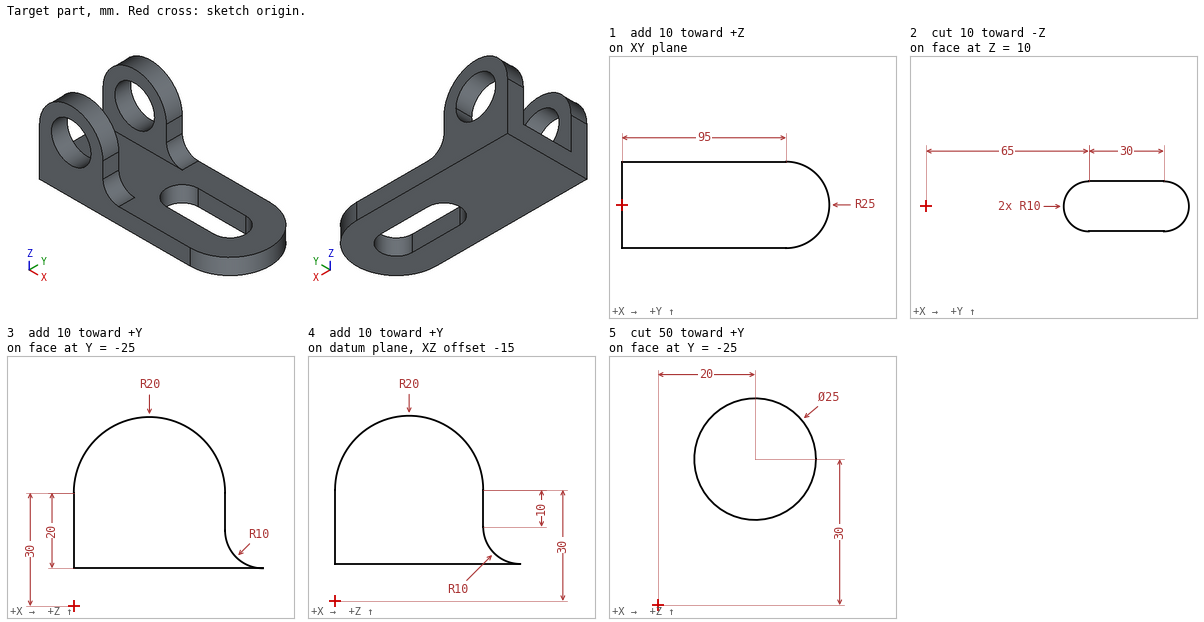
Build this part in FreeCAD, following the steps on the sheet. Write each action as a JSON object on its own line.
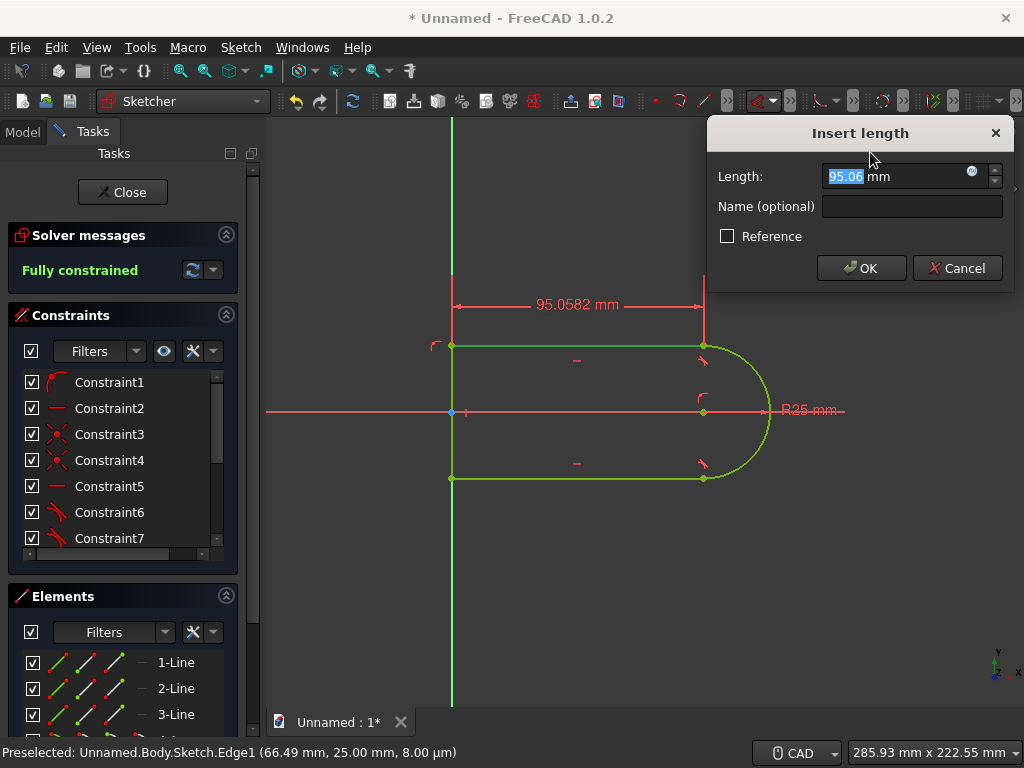
{"action": "type", "text": "95"}
{"action": "key", "text": "Return"}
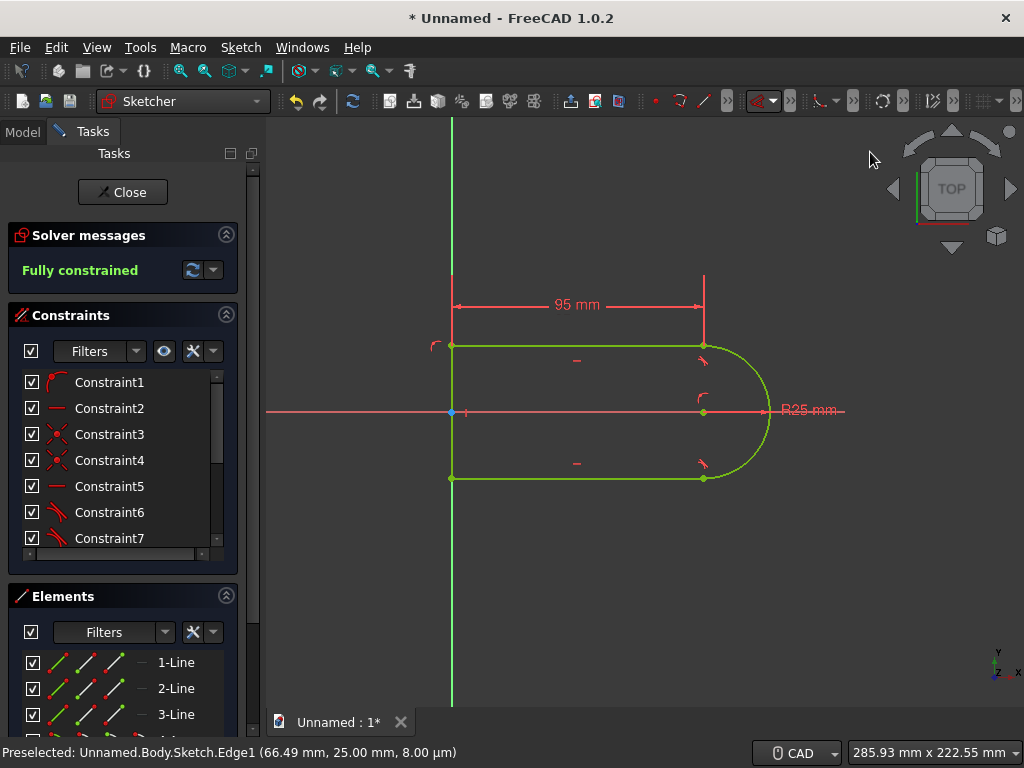
{"action": "left_click", "coordinate": [123, 192]}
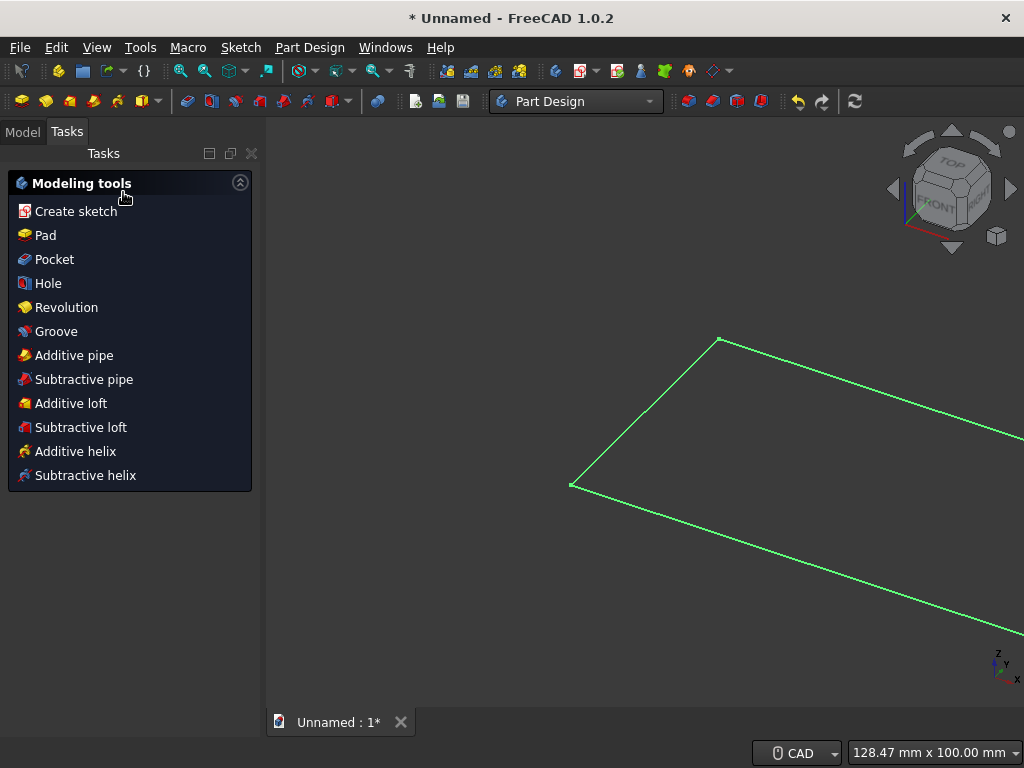
{"action": "left_click", "coordinate": [22, 102]}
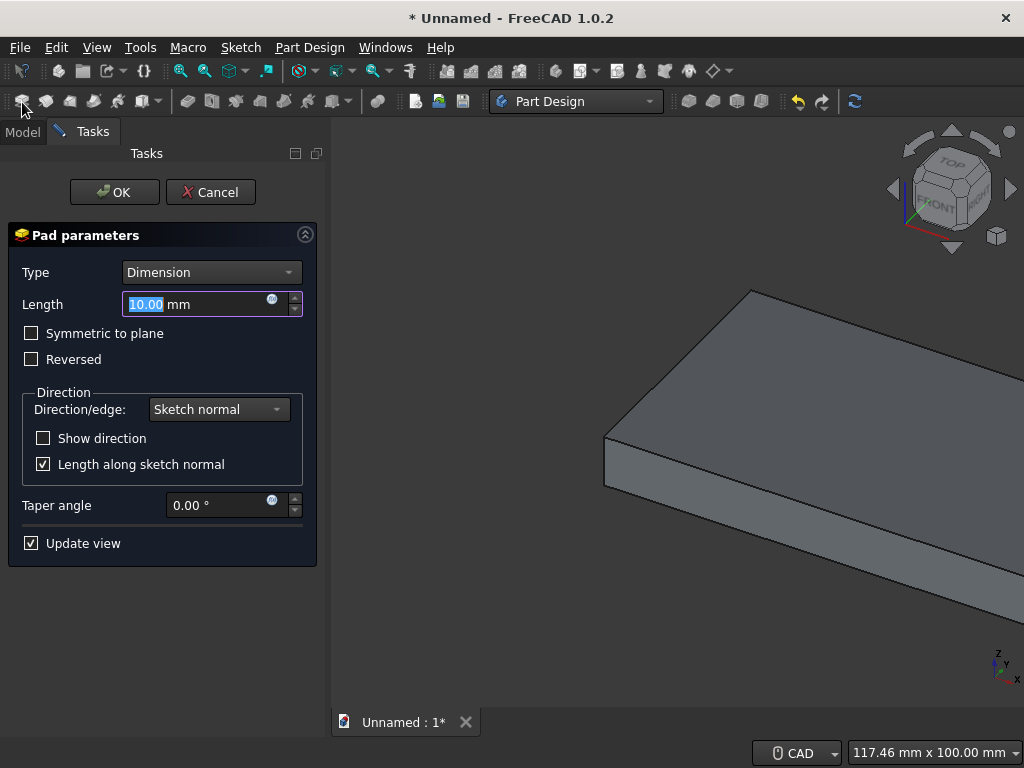
{"action": "type", "text": "10"}
{"action": "key", "text": "Tab"}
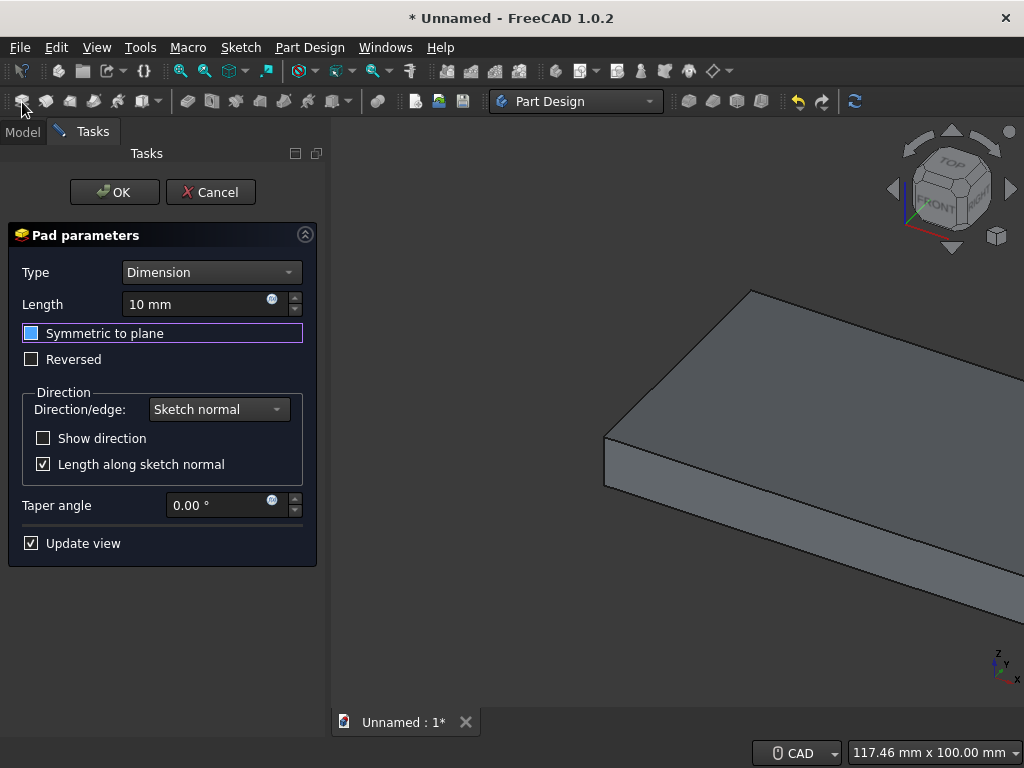
{"action": "left_click", "coordinate": [115, 192]}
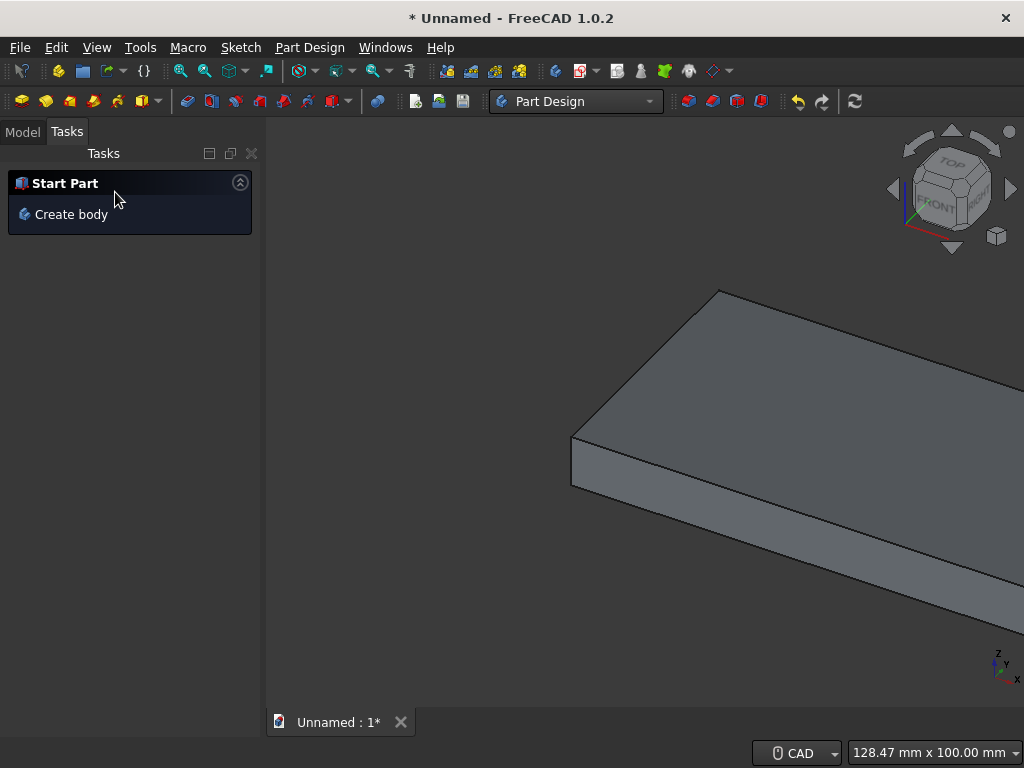
{"action": "left_click", "coordinate": [182, 72]}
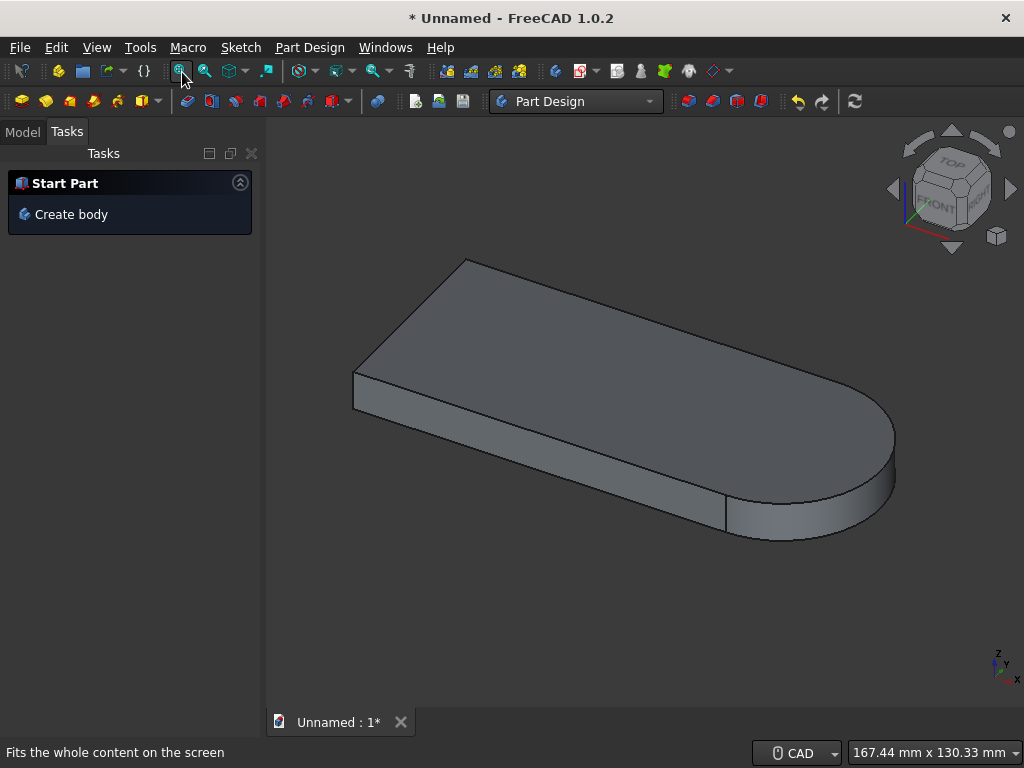
{"action": "left_click", "coordinate": [780, 437]}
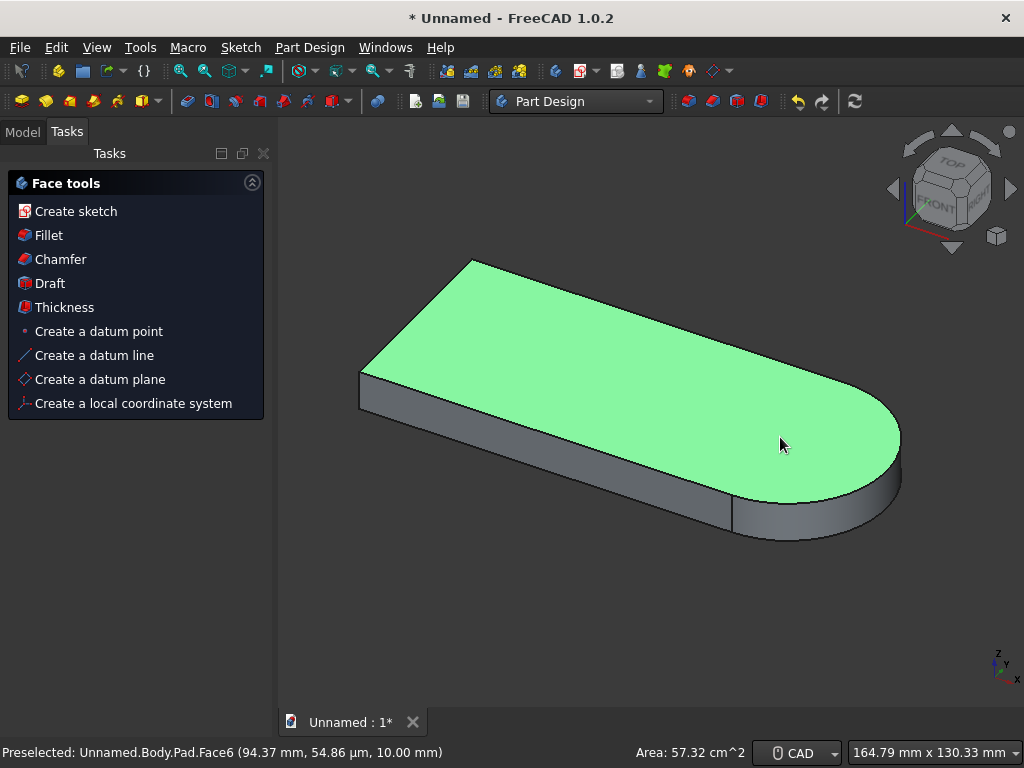
{"action": "left_click", "coordinate": [580, 72]}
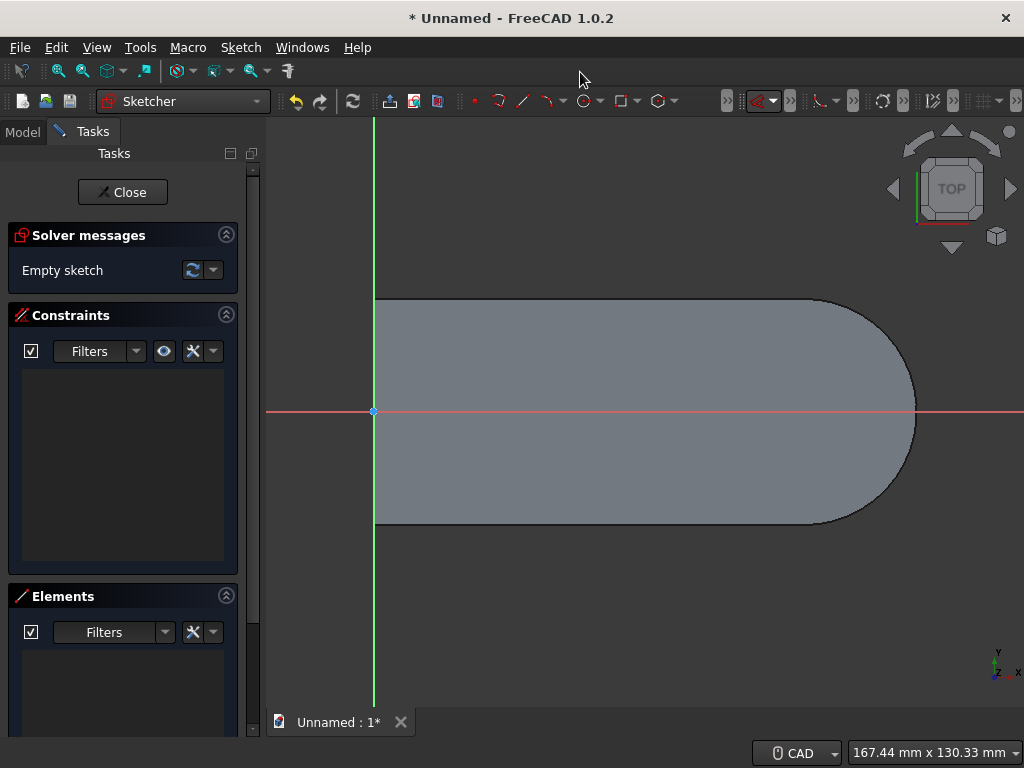
{"action": "scroll", "coordinate": [420, 412], "scroll_direction": "down", "scroll_amount": 1}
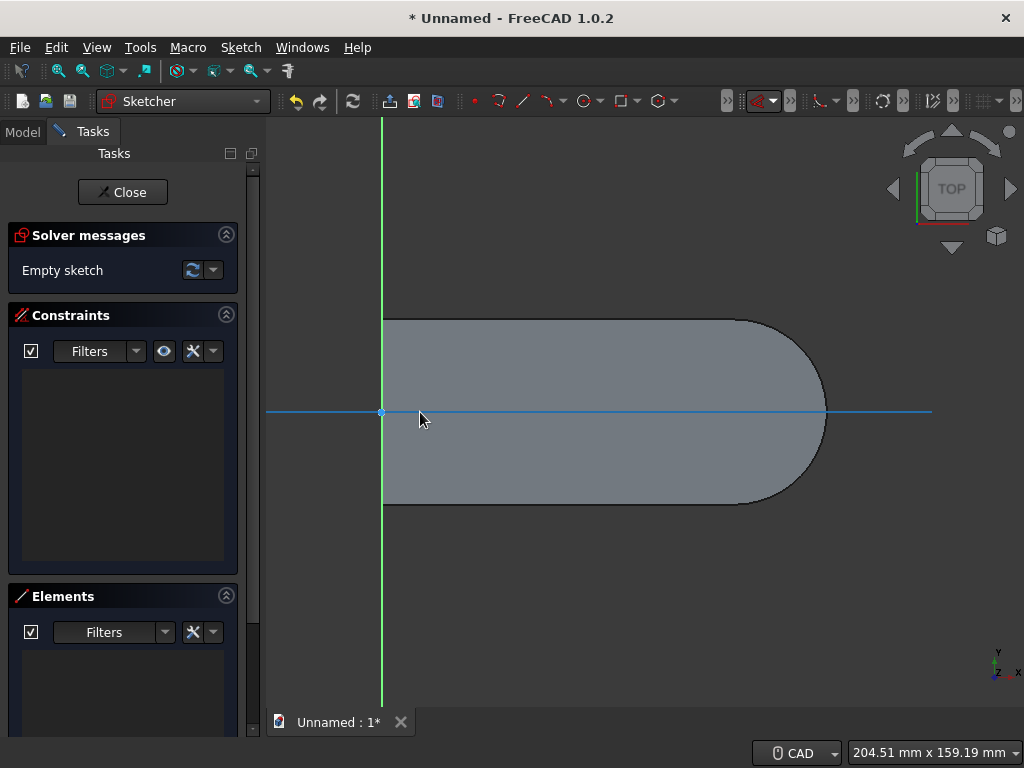
{"action": "key", "text": "g s"}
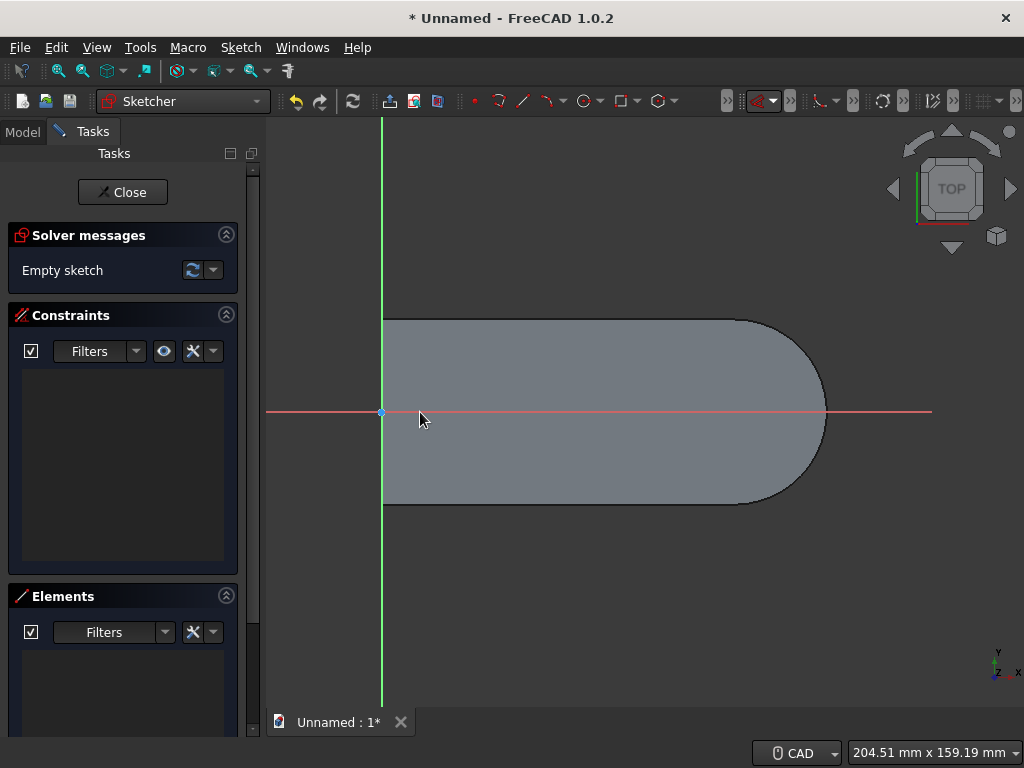
{"action": "left_click", "coordinate": [623, 412]}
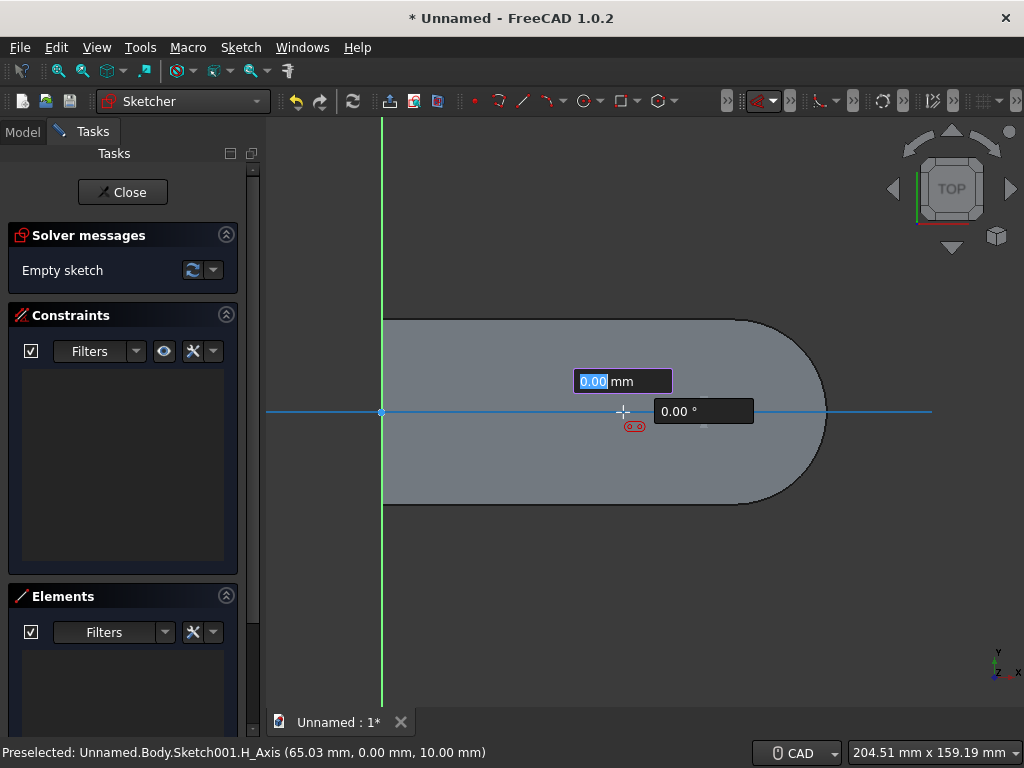
{"action": "left_click", "coordinate": [734, 403]}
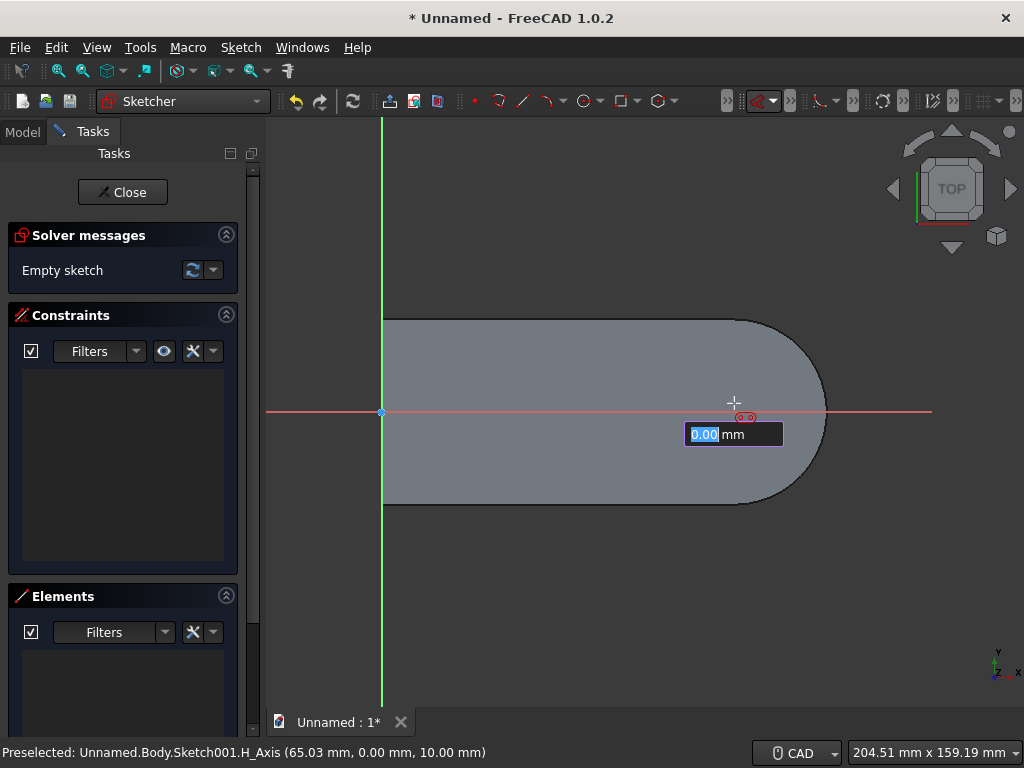
{"action": "left_click", "coordinate": [678, 375]}
{"action": "key", "text": "Escape"}